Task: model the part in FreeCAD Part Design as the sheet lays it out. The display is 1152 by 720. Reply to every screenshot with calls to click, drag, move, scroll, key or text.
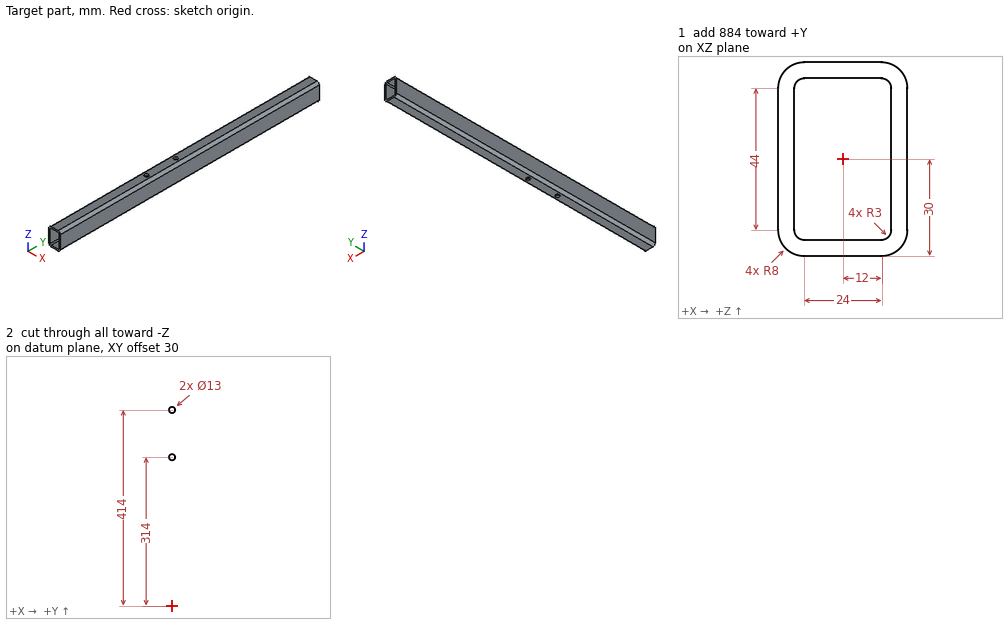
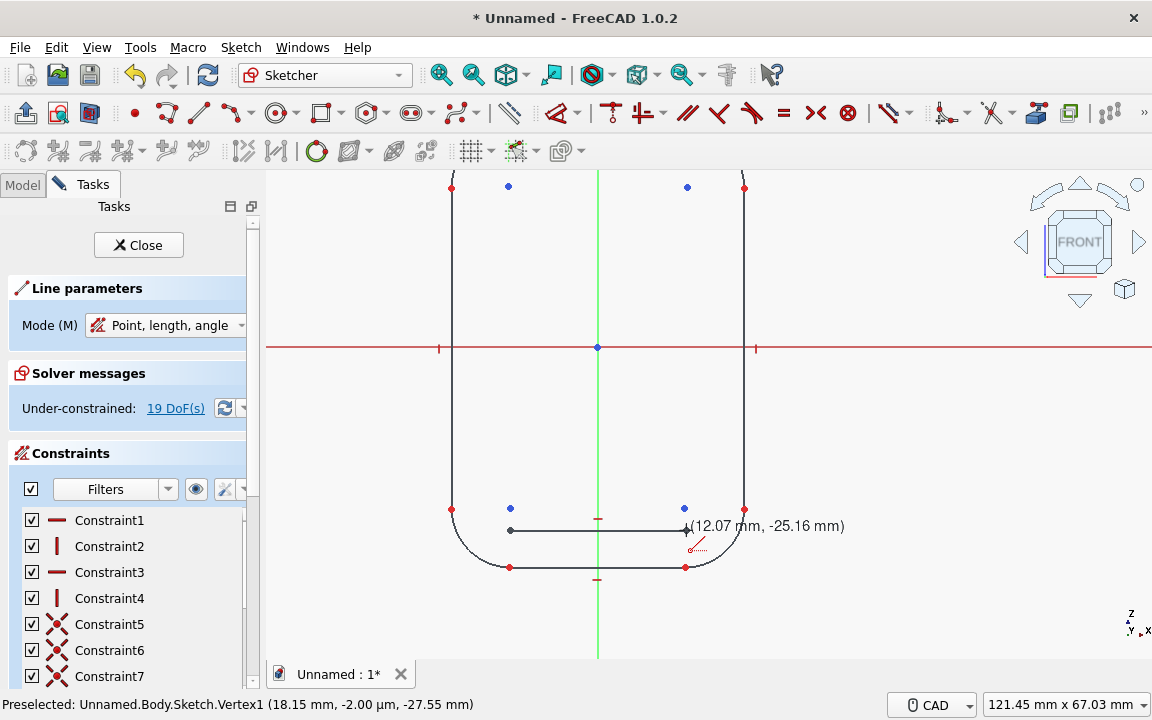
click(707, 508)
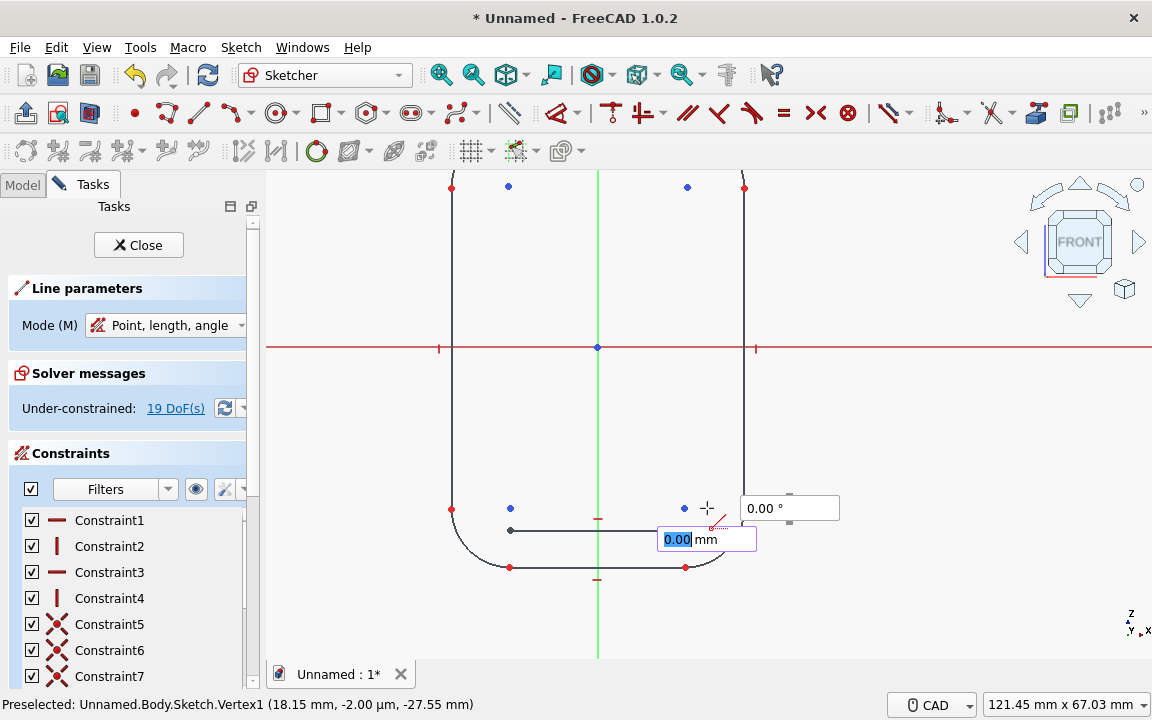
scroll(727, 551, down, 2)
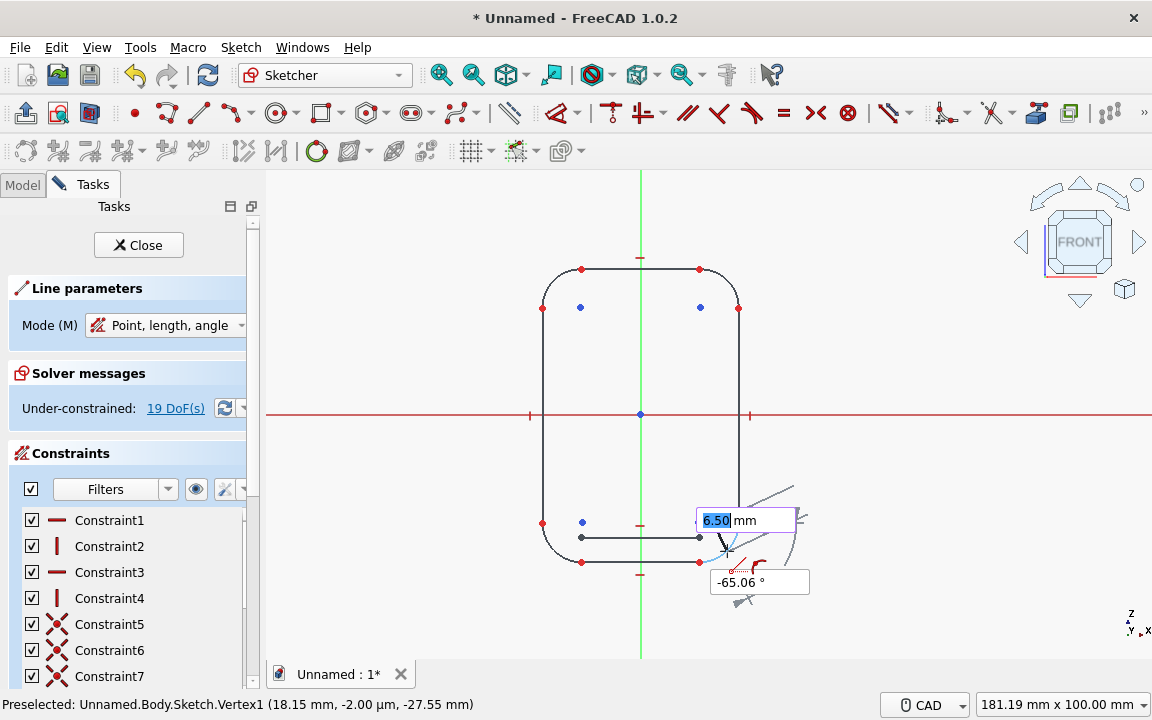
click(714, 307)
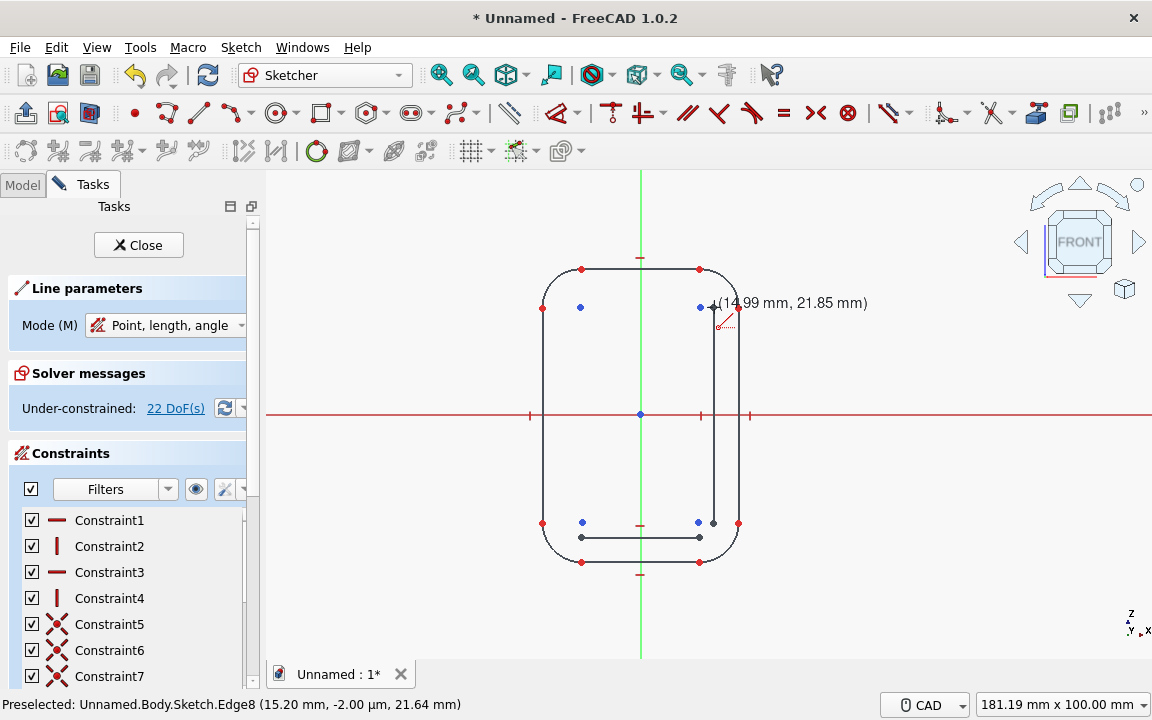
click(699, 293)
click(582, 293)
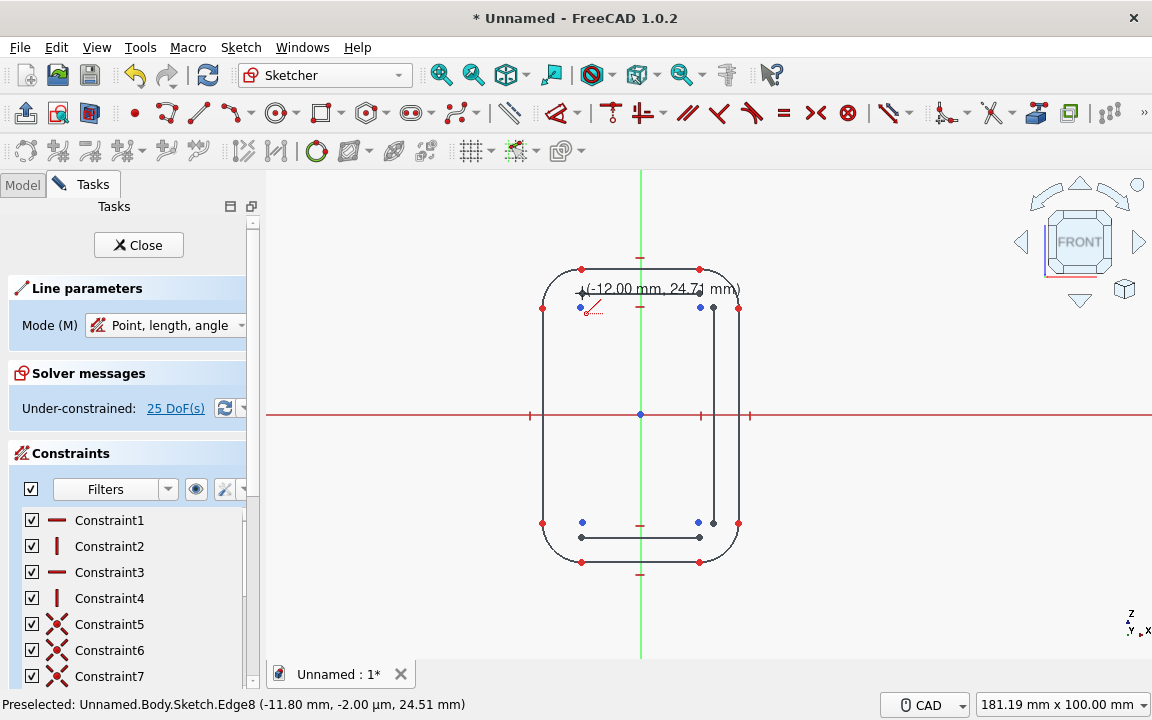
click(567, 307)
click(567, 522)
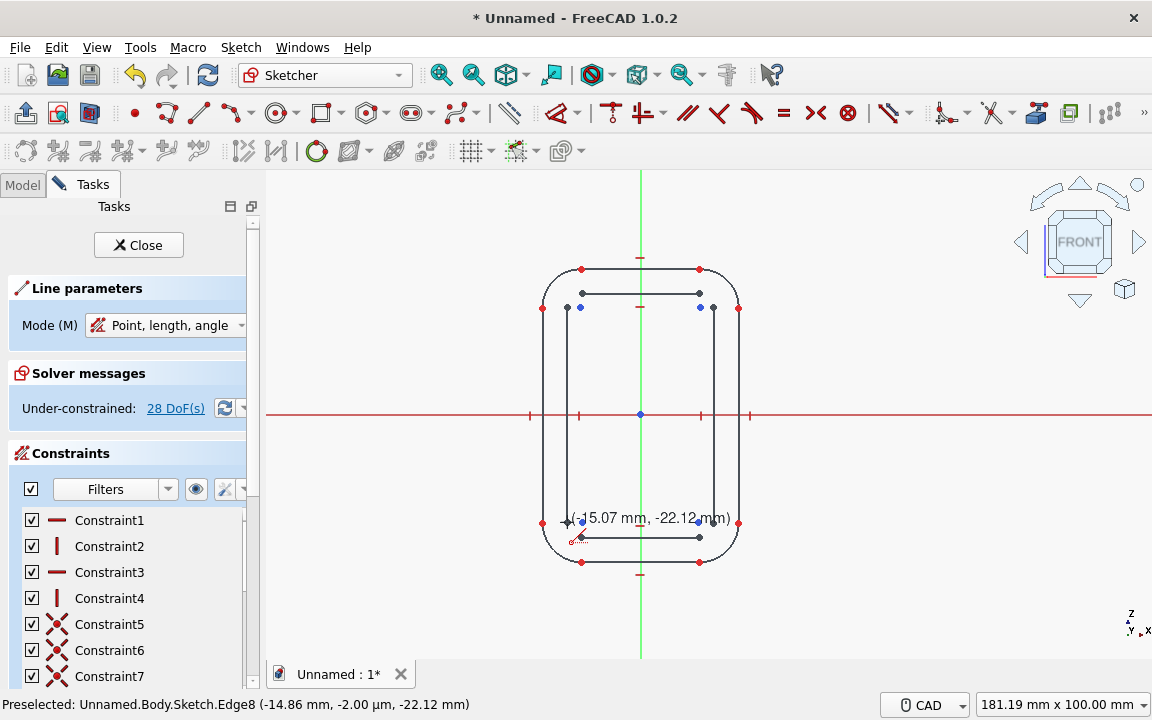
key(g)
key(3)
key(a)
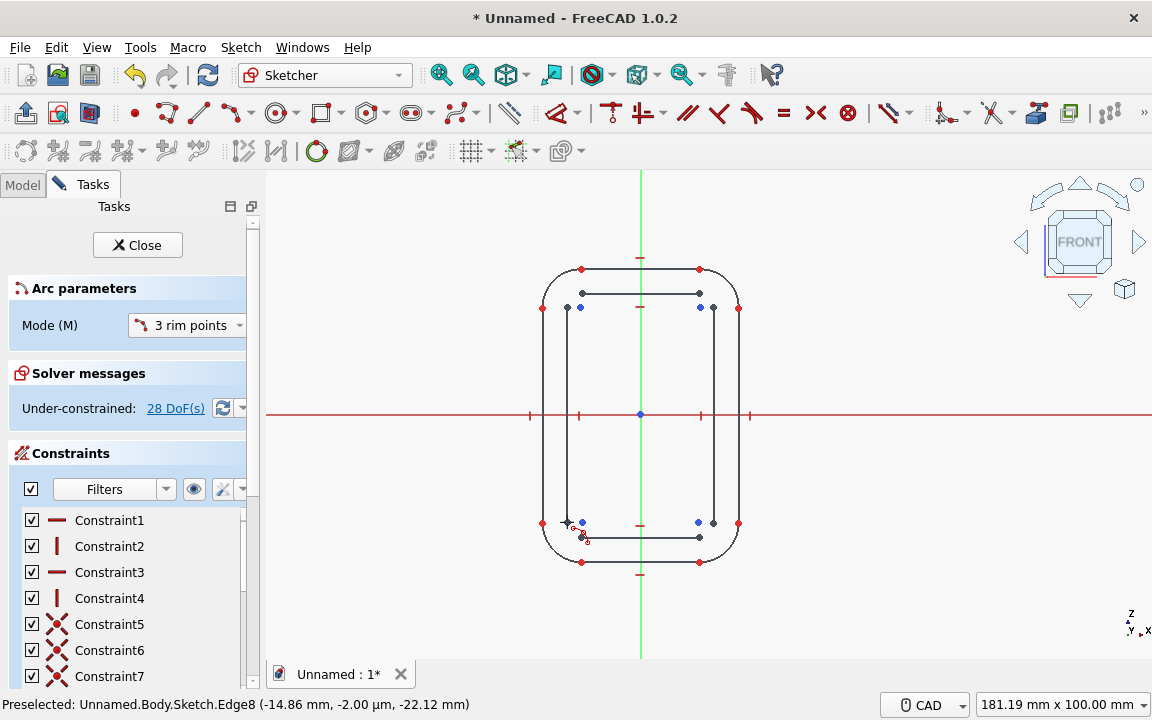
click(700, 538)
click(714, 523)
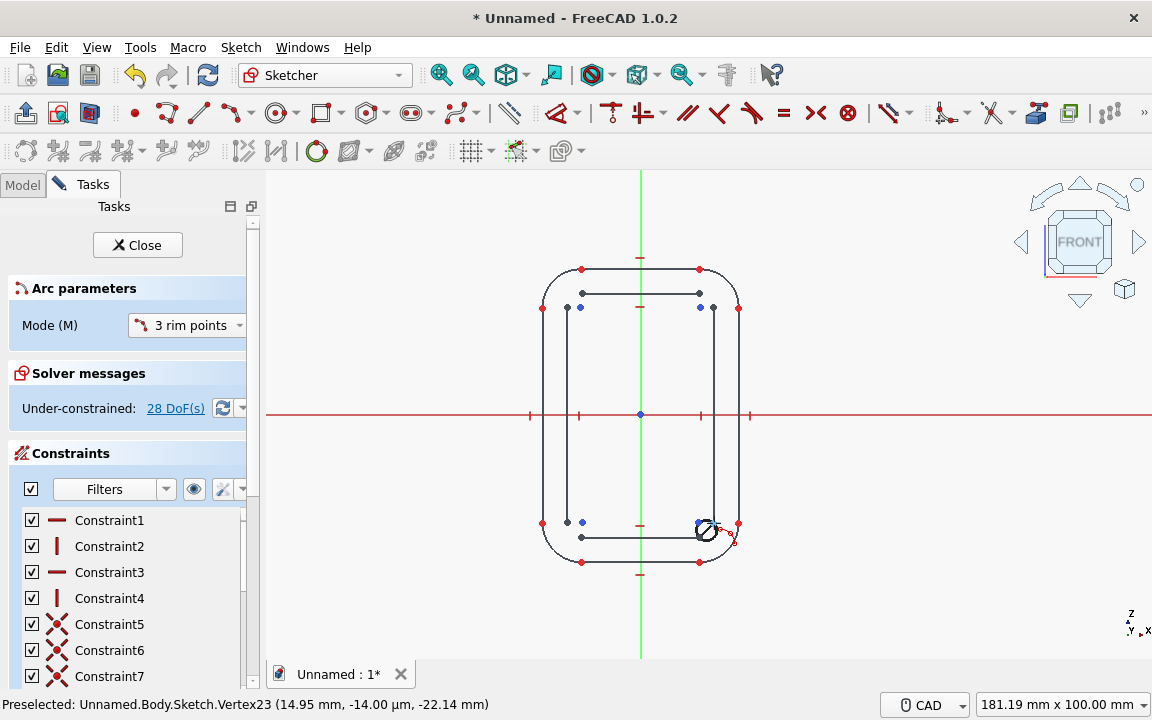
scroll(710, 533, up, 7)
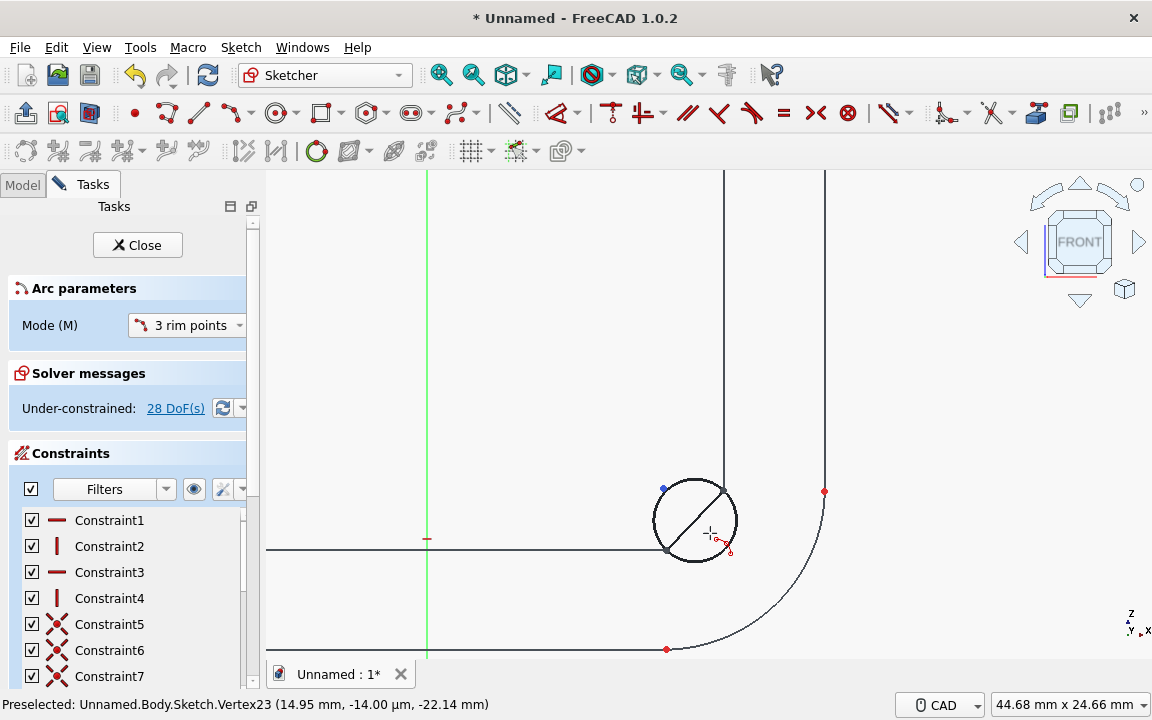
click(707, 530)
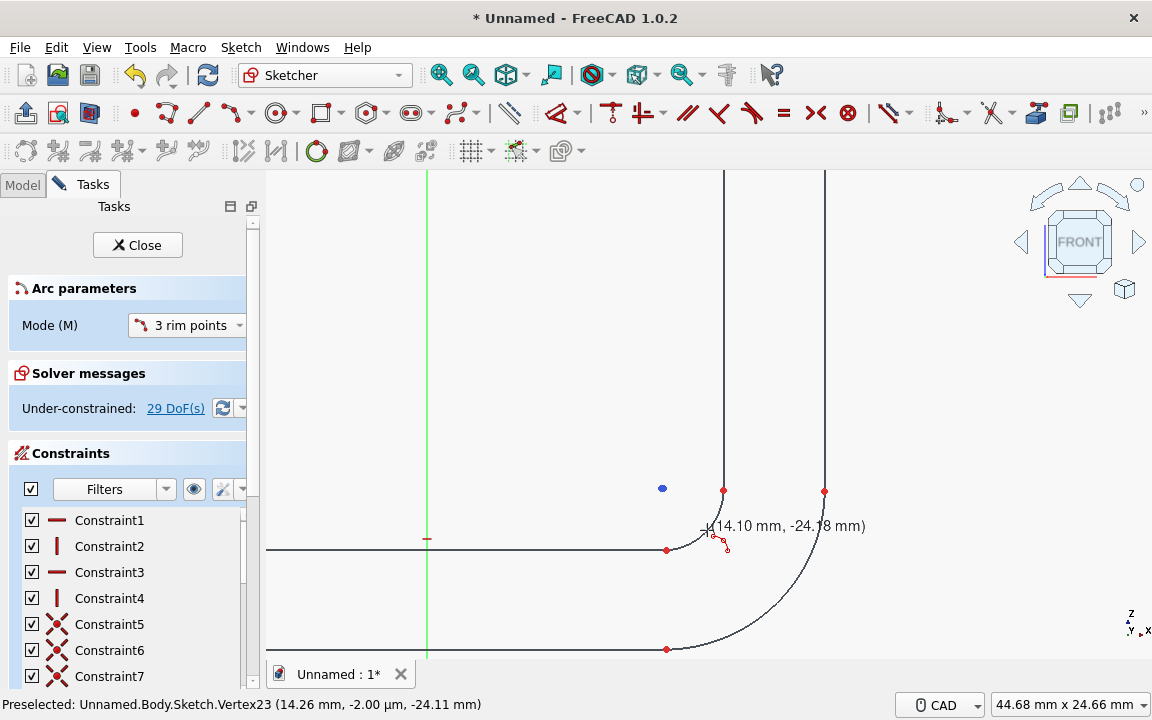
scroll(710, 533, down, 7)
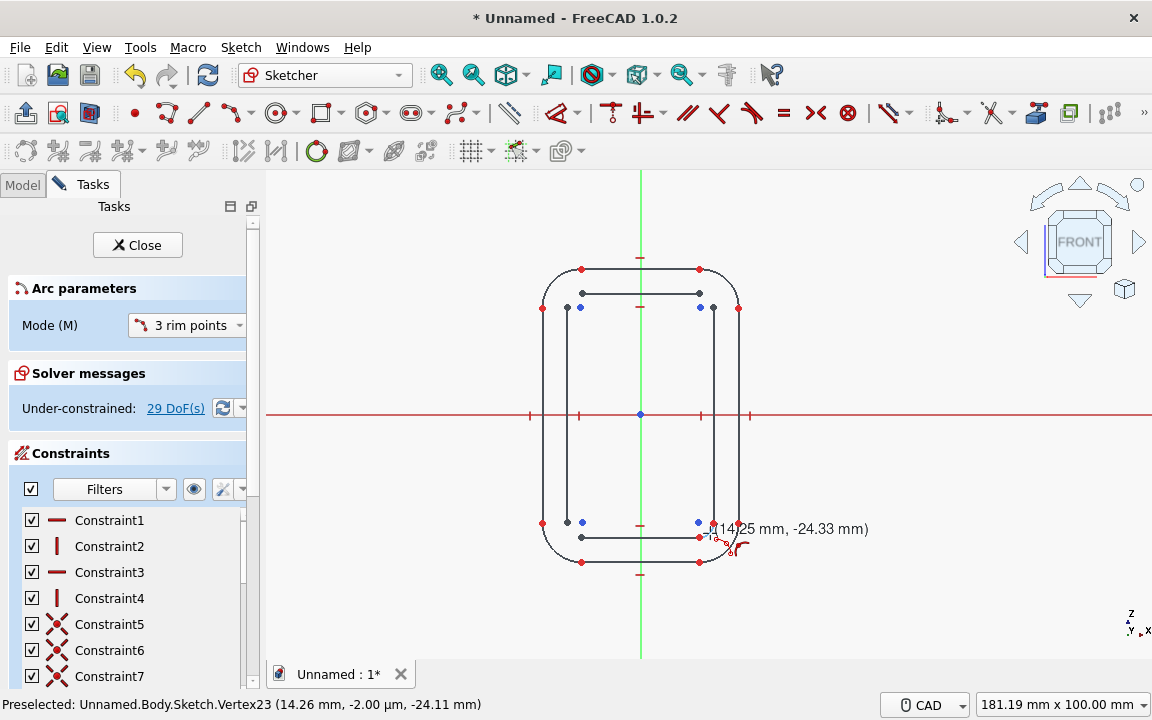
click(714, 308)
click(699, 294)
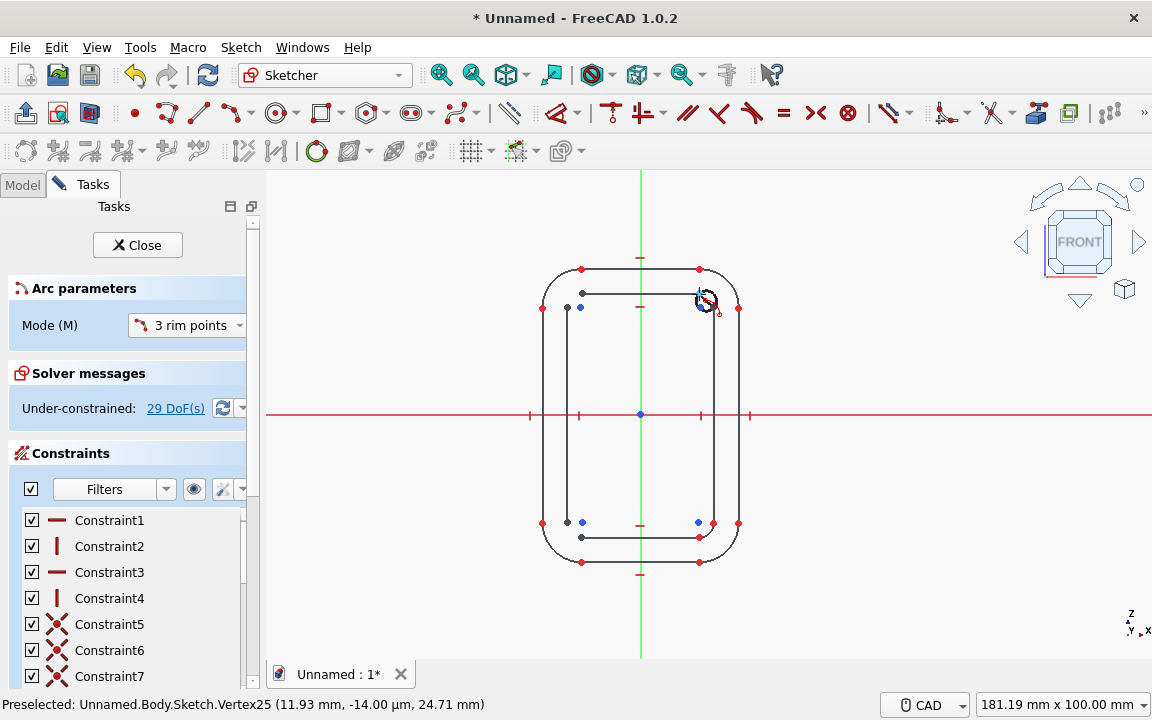
scroll(710, 297, up, 7)